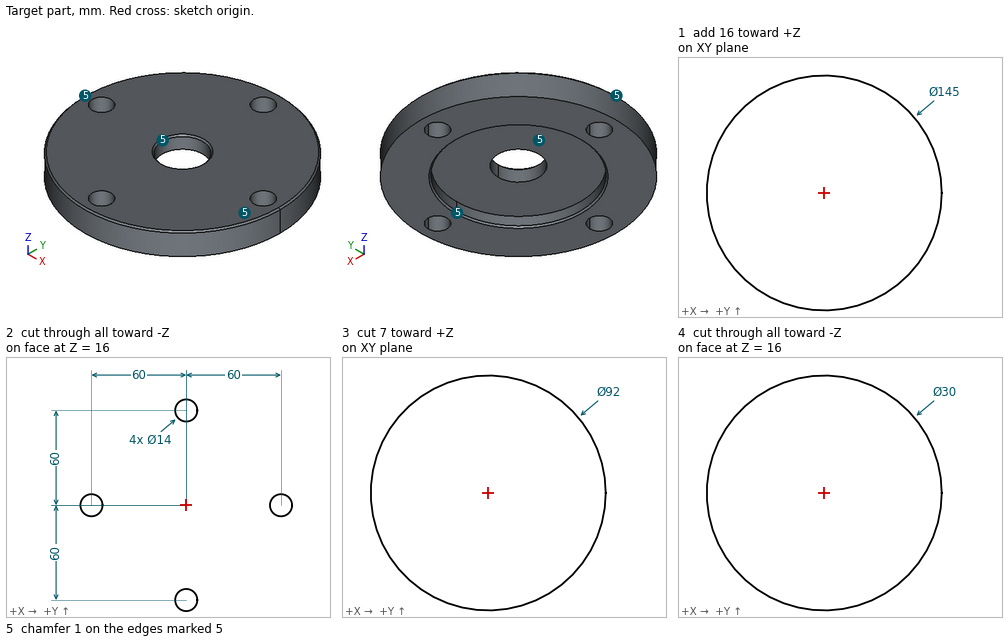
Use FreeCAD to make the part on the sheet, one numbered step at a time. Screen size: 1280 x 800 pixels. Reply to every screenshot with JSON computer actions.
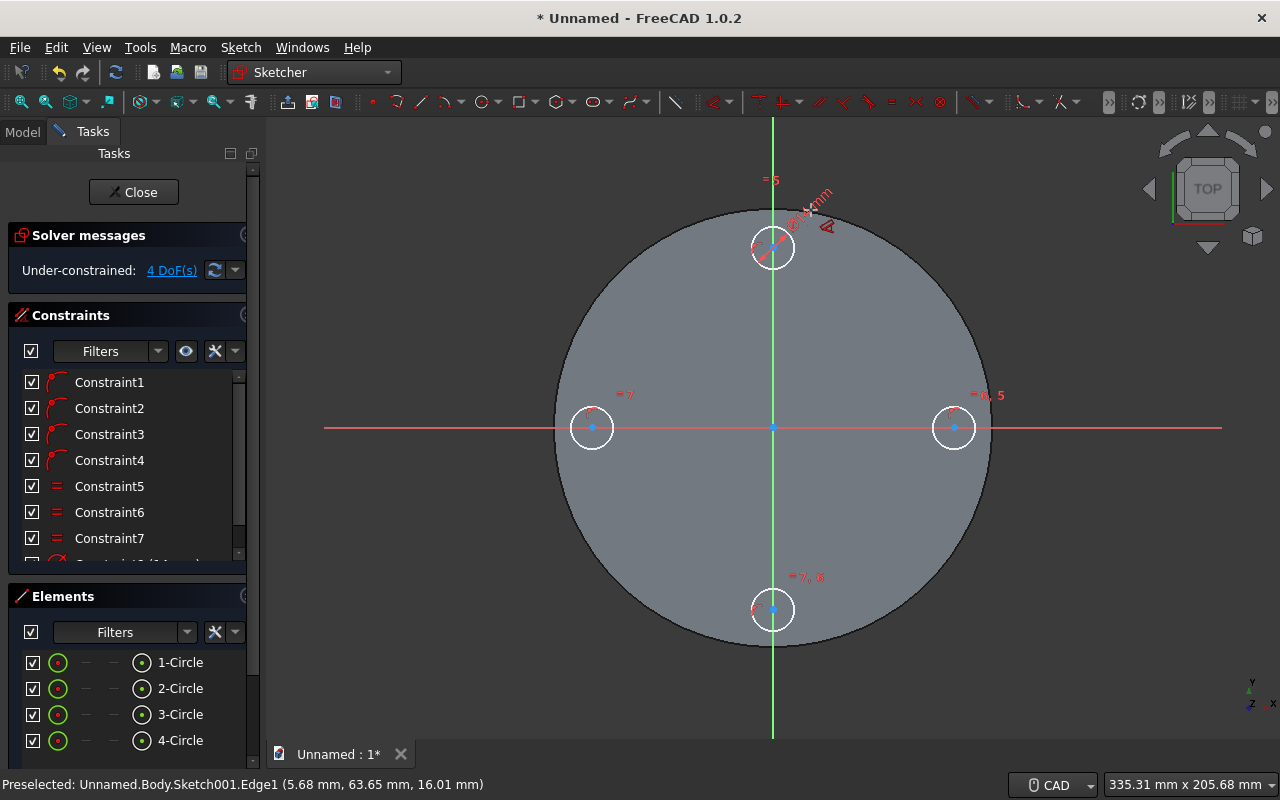
{"action": "left_click", "coordinate": [773, 248]}
{"action": "left_click", "coordinate": [807, 338]}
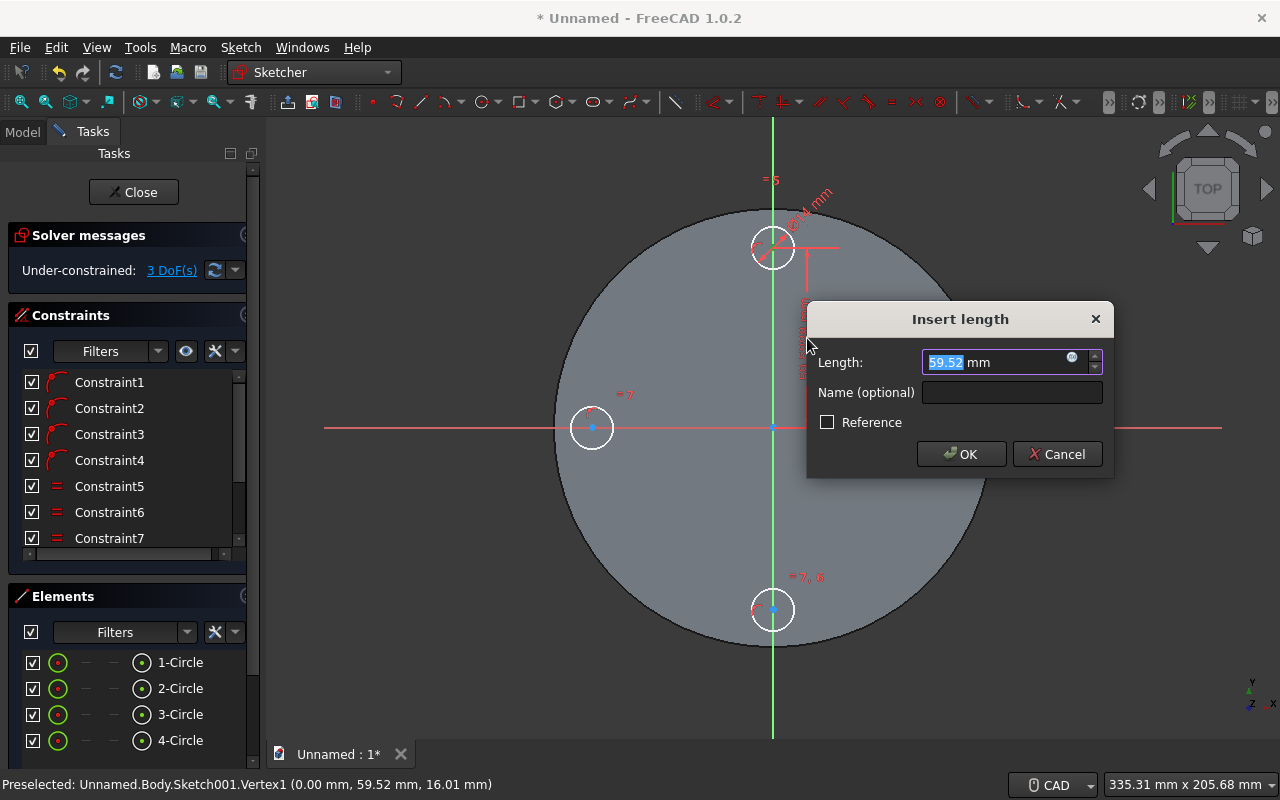
{"action": "type", "text": "60"}
{"action": "key", "text": "Return"}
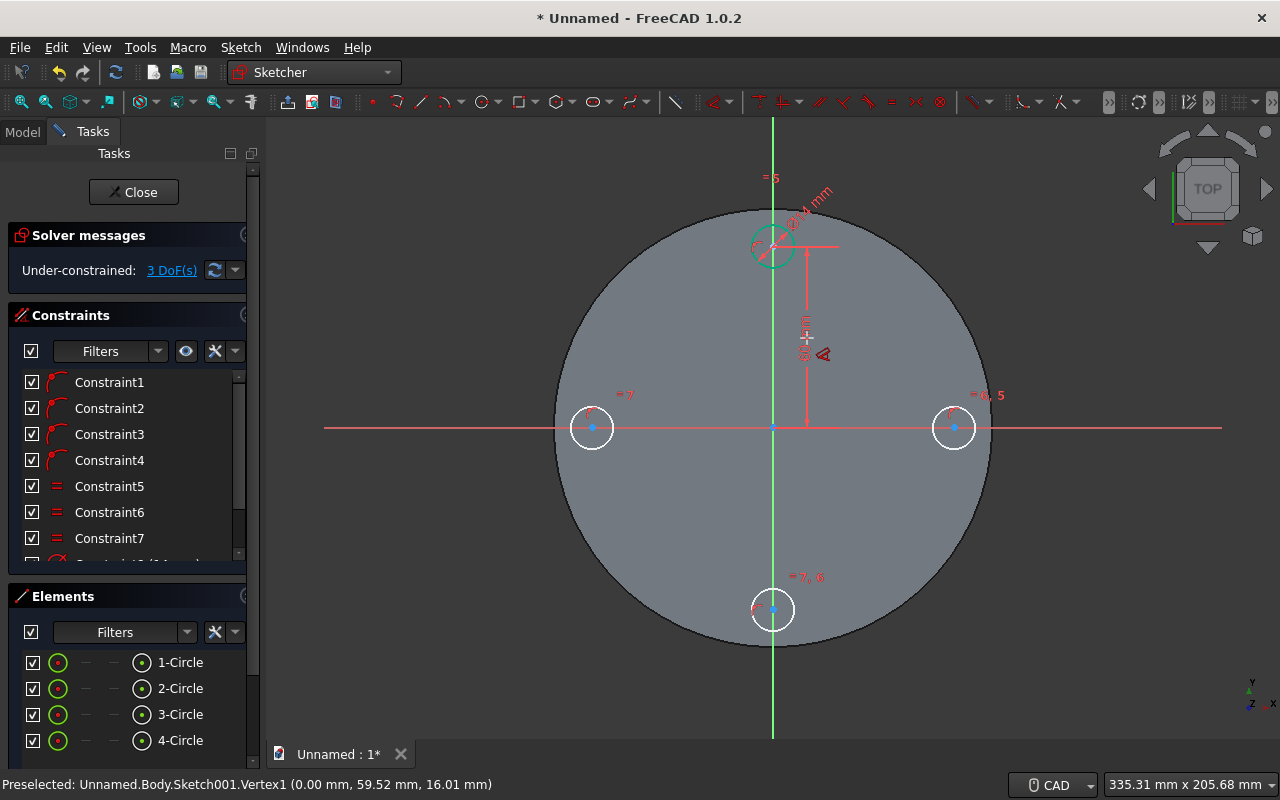
{"action": "left_click", "coordinate": [954, 428]}
{"action": "left_click", "coordinate": [864, 462]}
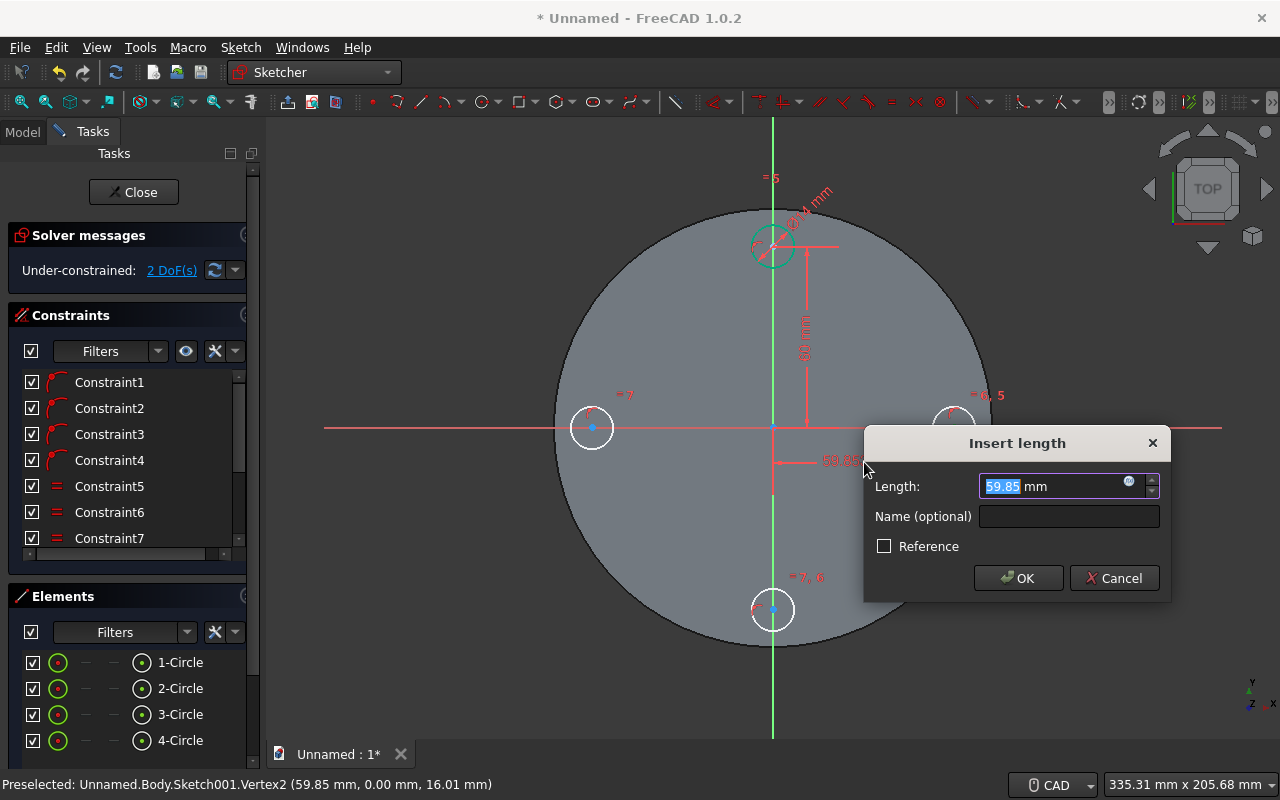
{"action": "type", "text": "60"}
{"action": "key", "text": "Return"}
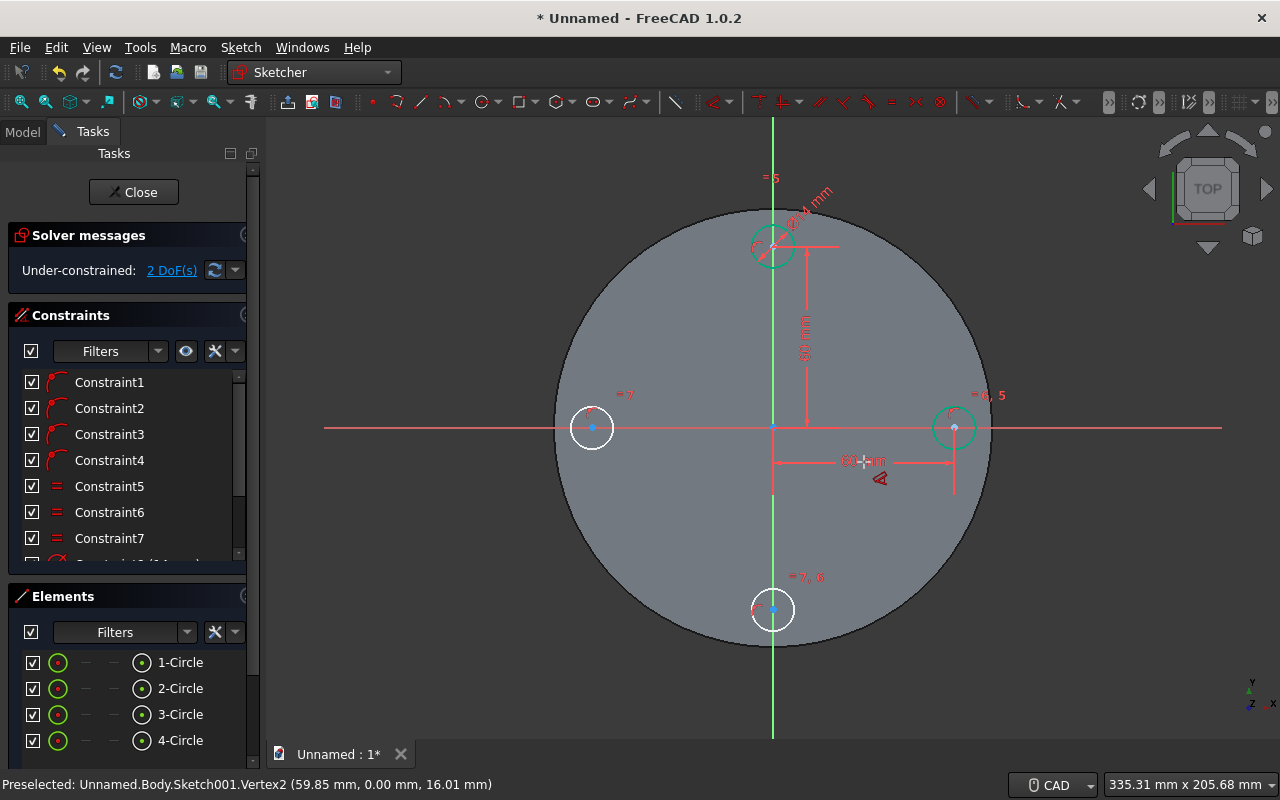
{"action": "left_click", "coordinate": [773, 610]}
{"action": "left_click", "coordinate": [807, 519]}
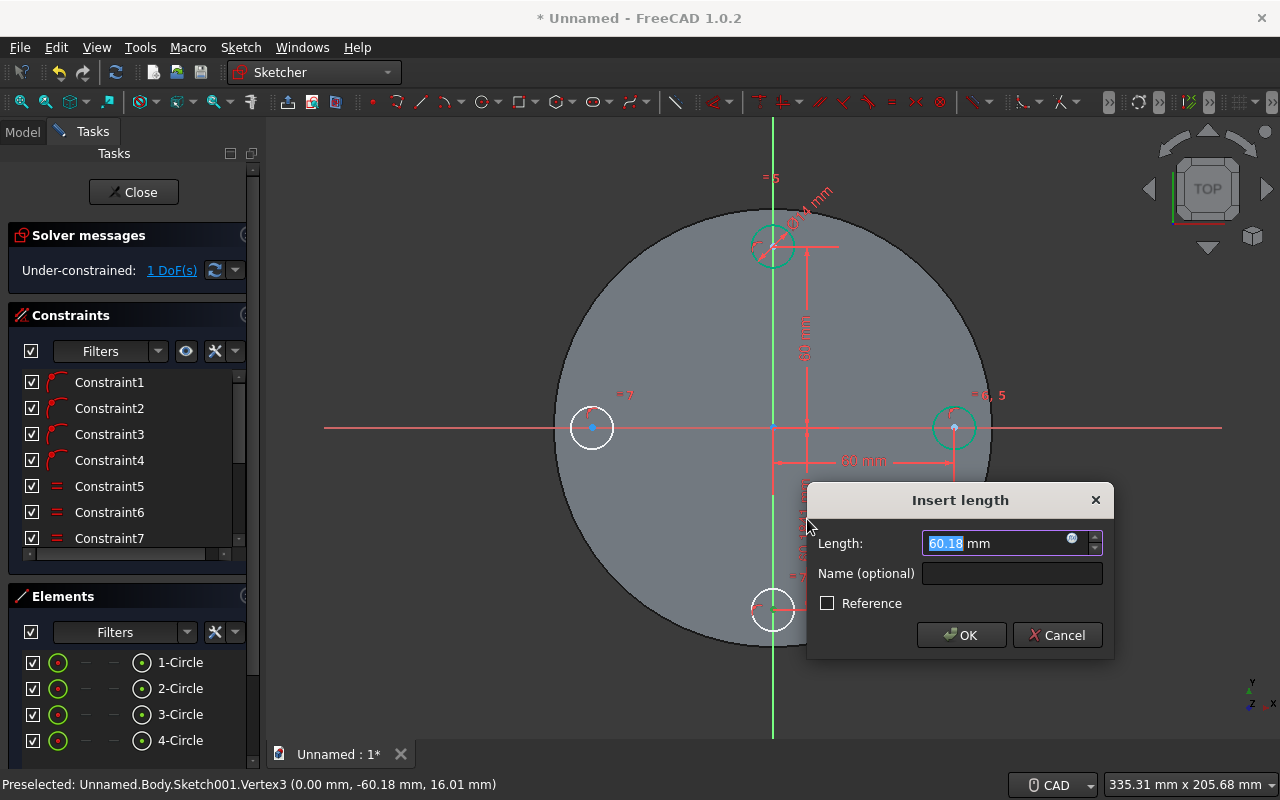
{"action": "type", "text": "60"}
{"action": "key", "text": "Return"}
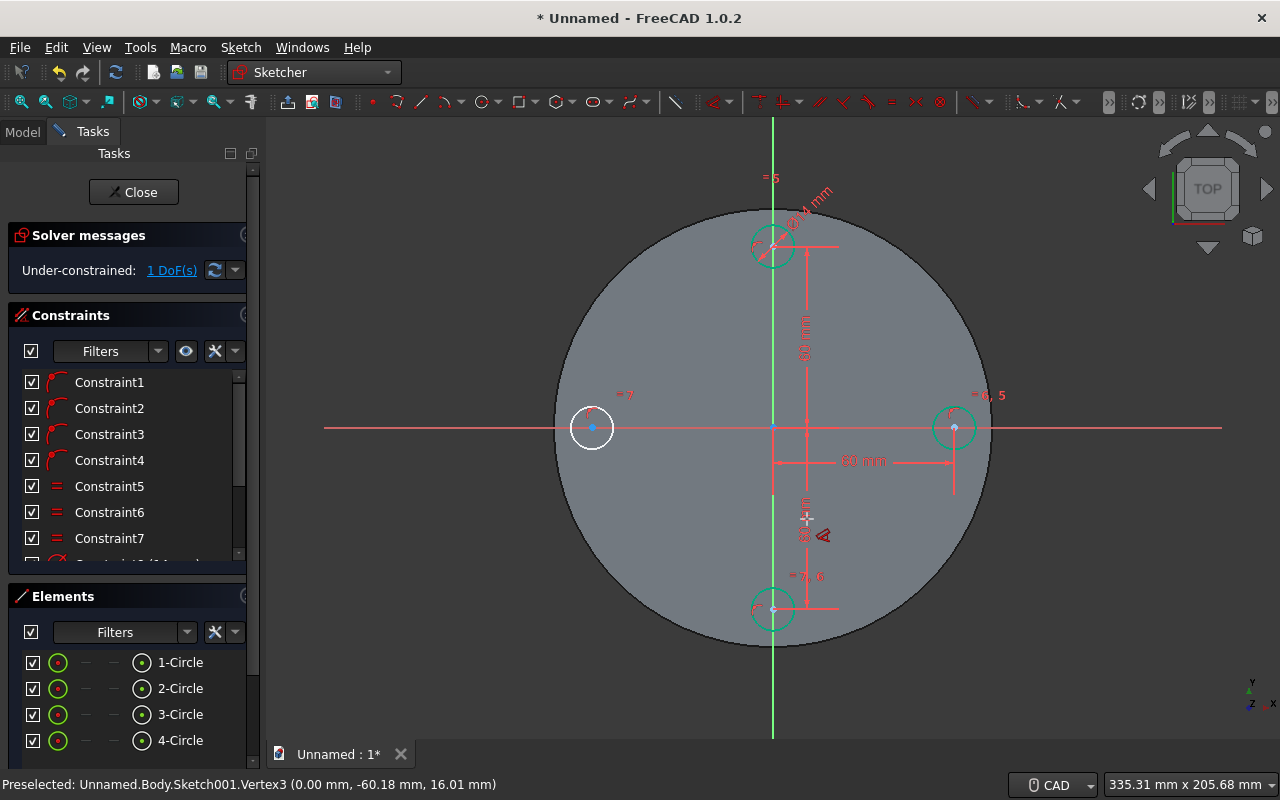
{"action": "left_click", "coordinate": [592, 428]}
{"action": "left_click", "coordinate": [683, 462]}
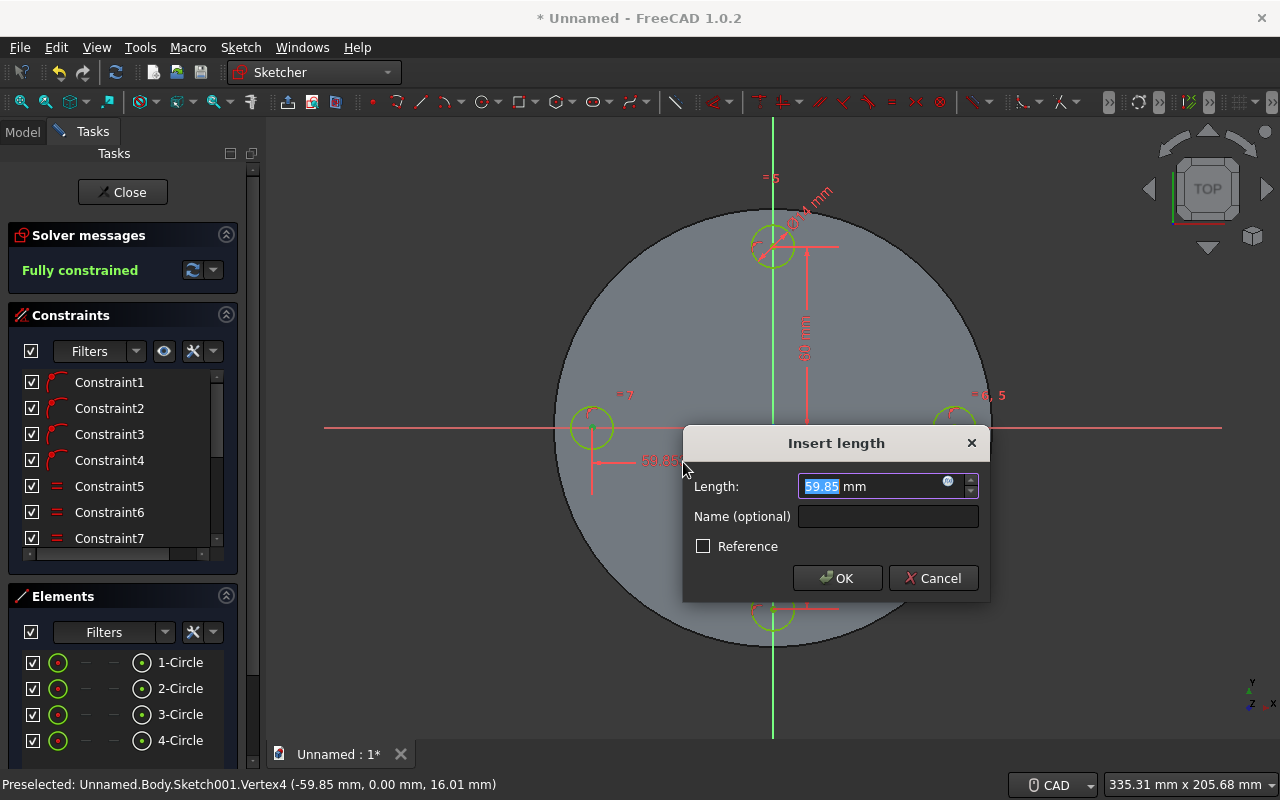
{"action": "type", "text": "60"}
{"action": "key", "text": "Return"}
{"action": "key", "text": "Escape"}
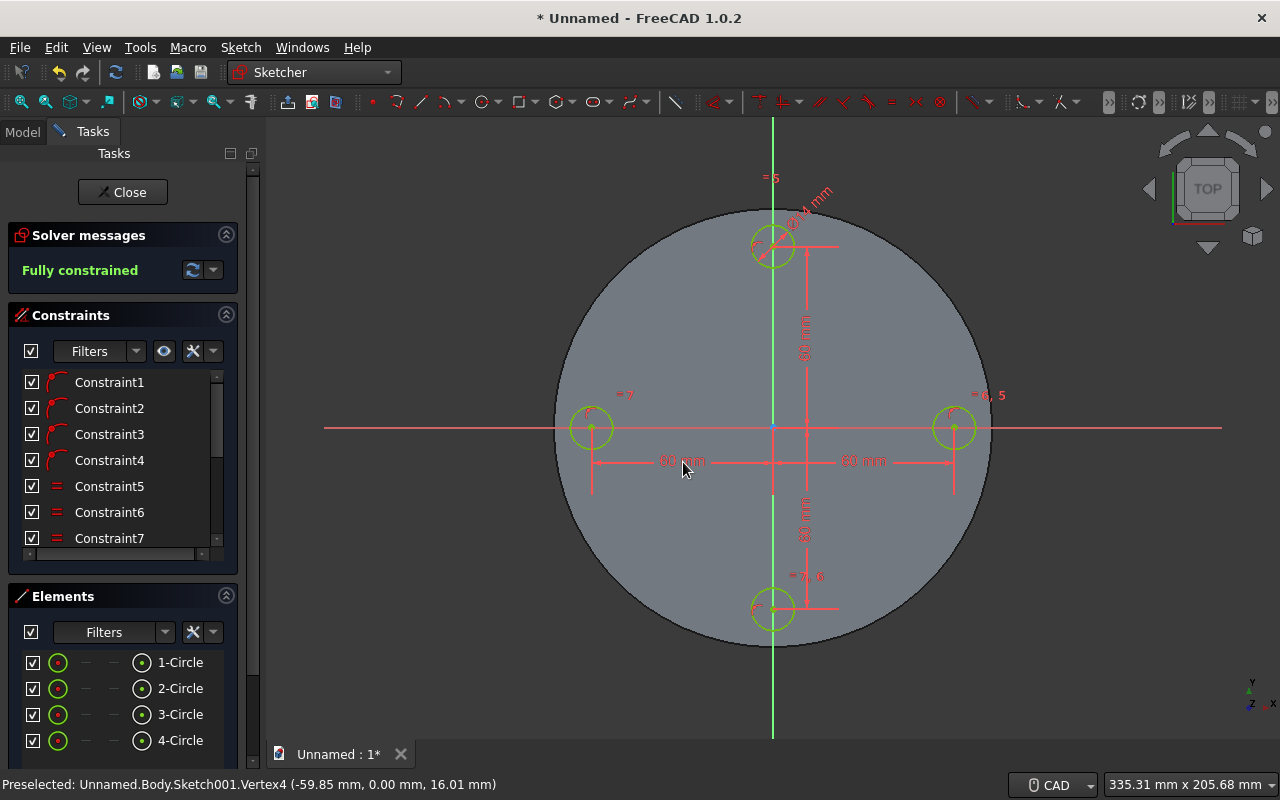
{"action": "left_click", "coordinate": [123, 192]}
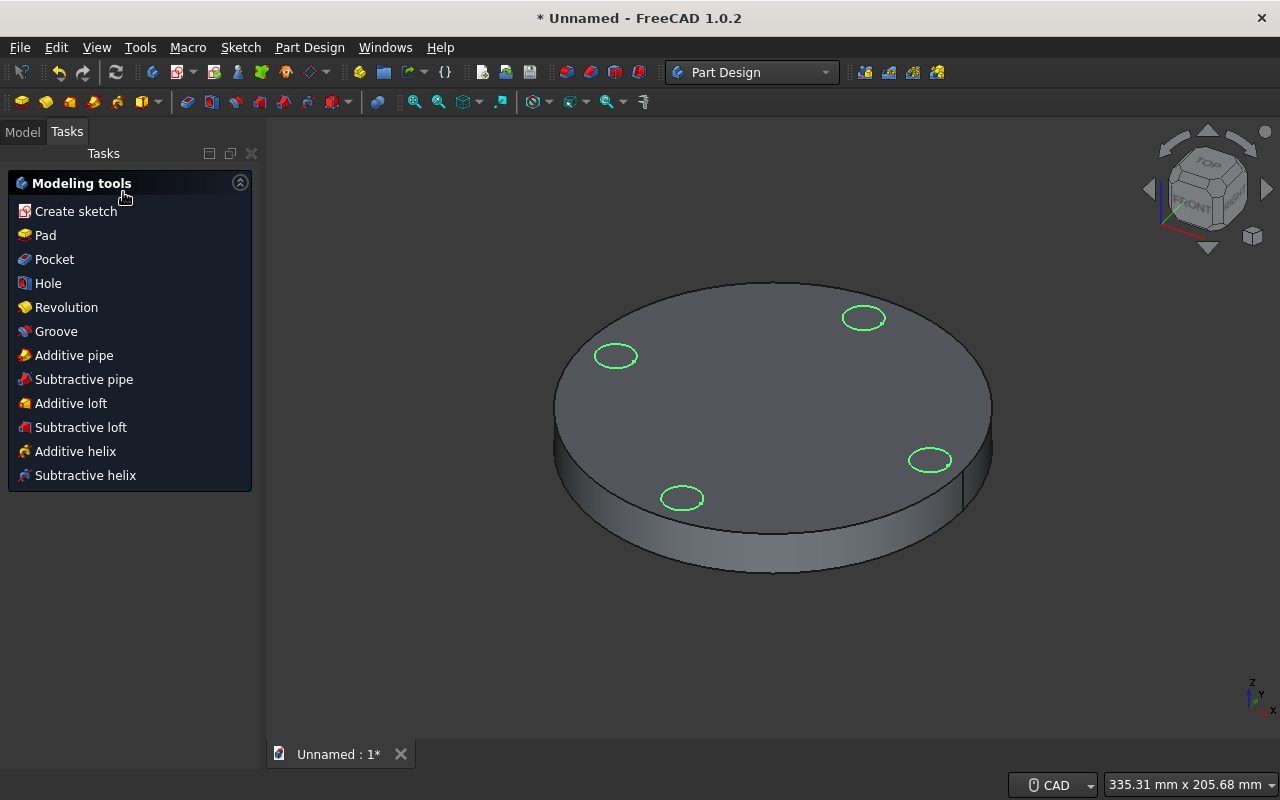
{"action": "left_click", "coordinate": [188, 102]}